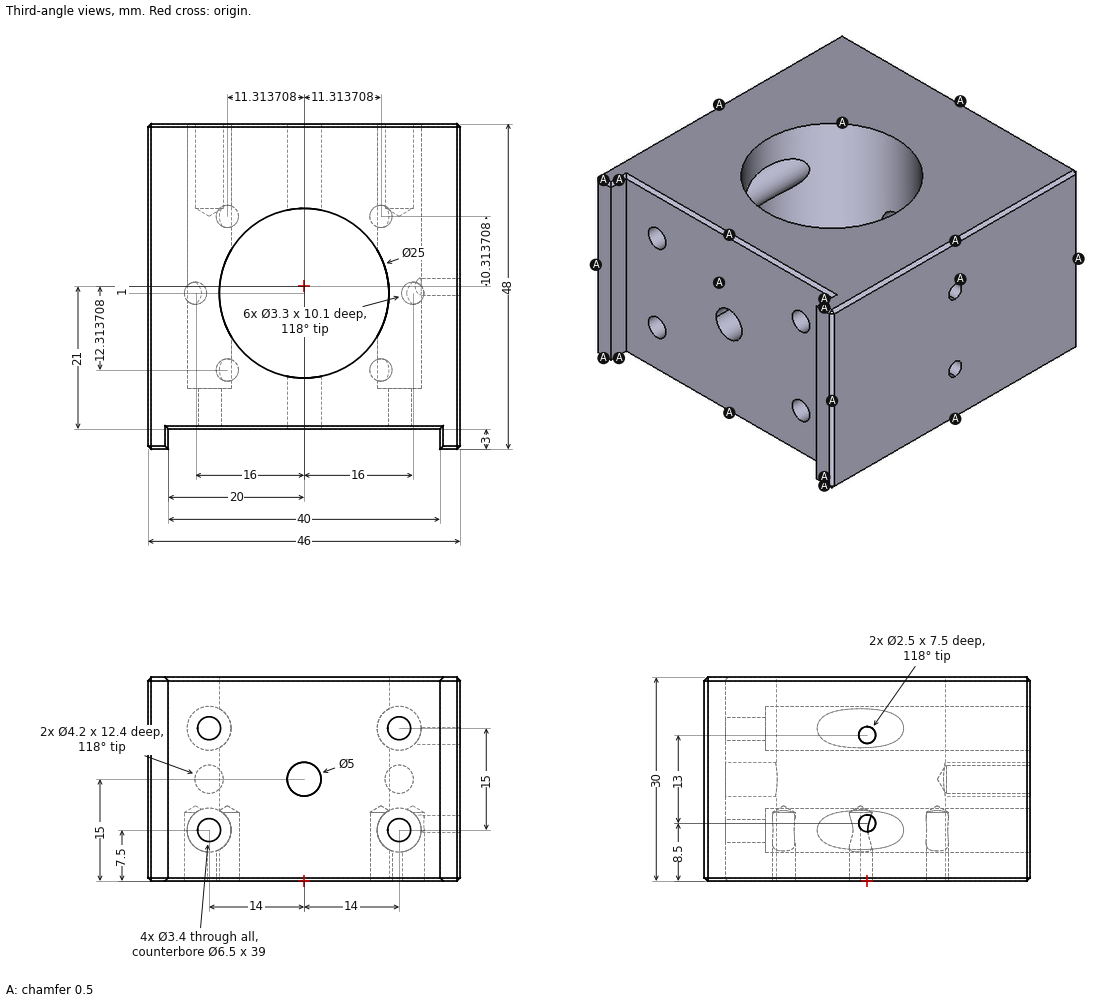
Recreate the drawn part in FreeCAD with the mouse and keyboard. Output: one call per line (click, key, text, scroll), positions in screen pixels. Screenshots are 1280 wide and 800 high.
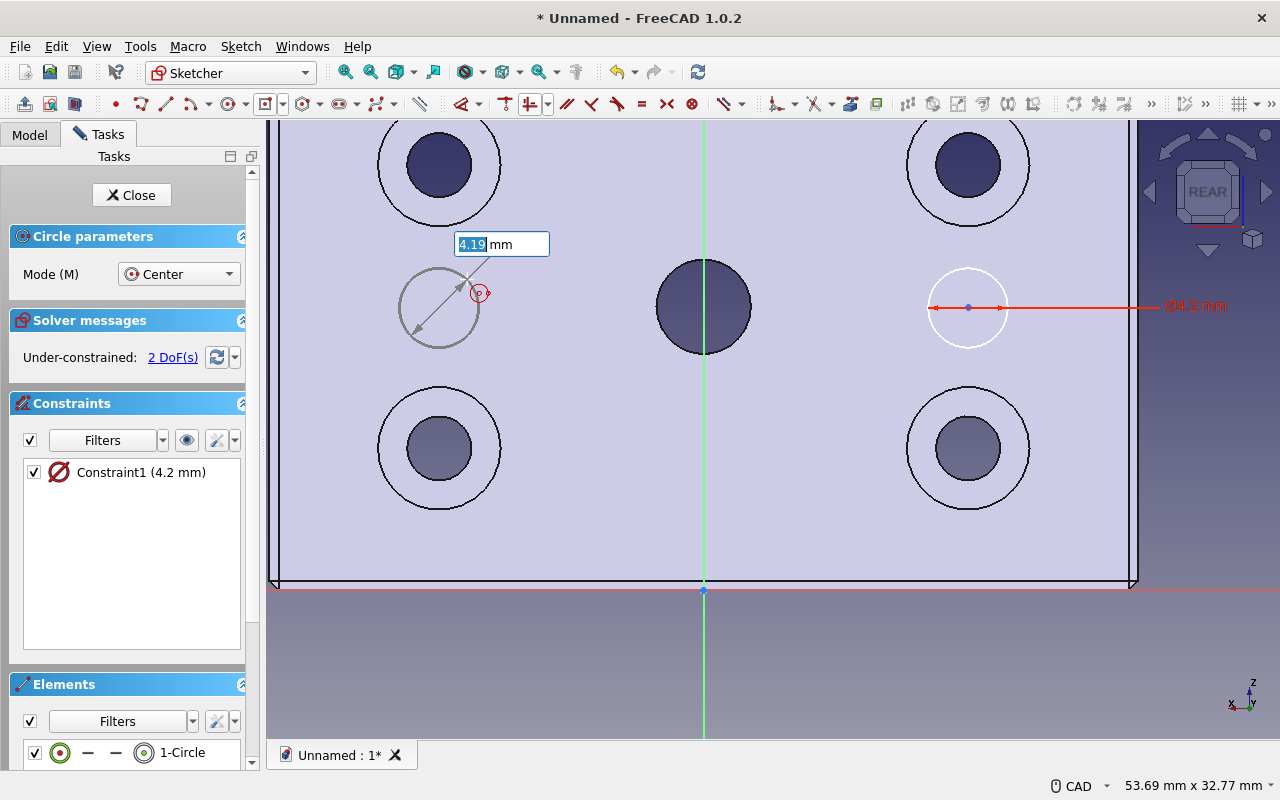
text(4.2)
key(Return)
key(Escape)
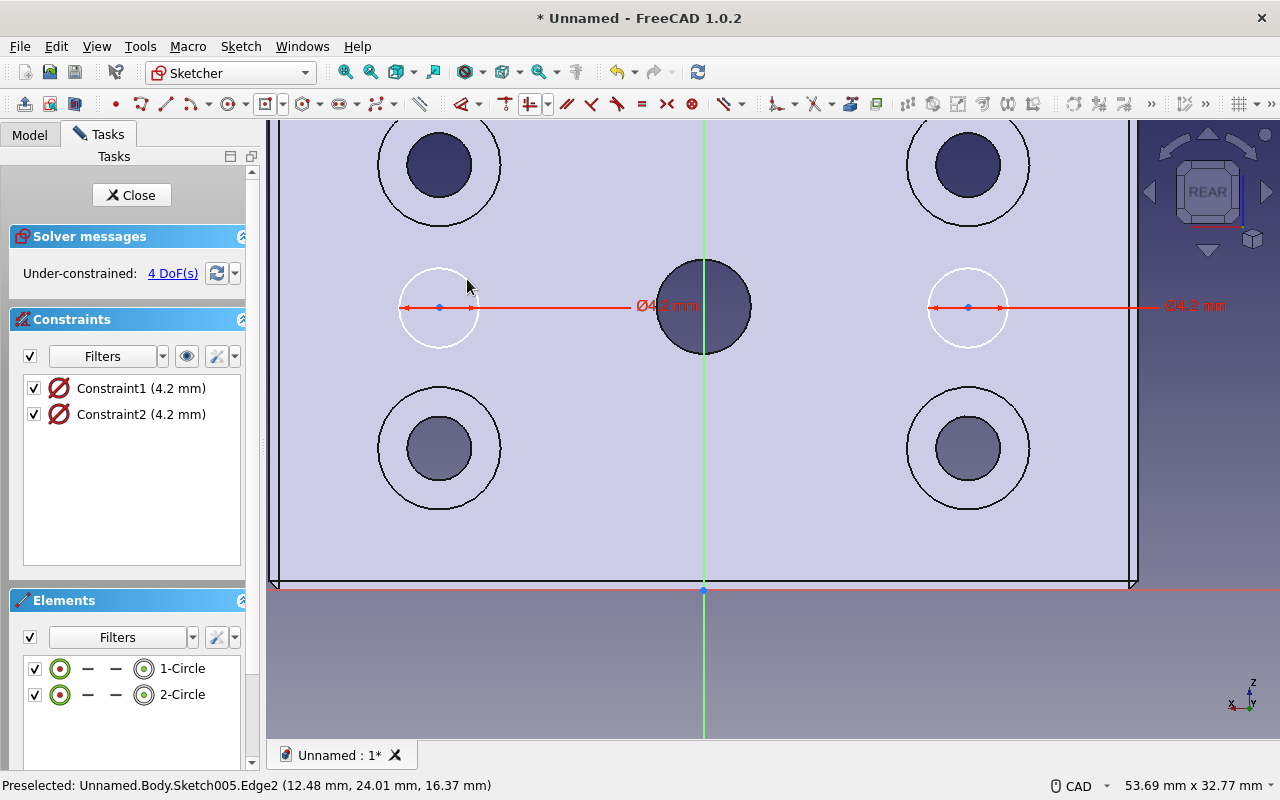
click(968, 308)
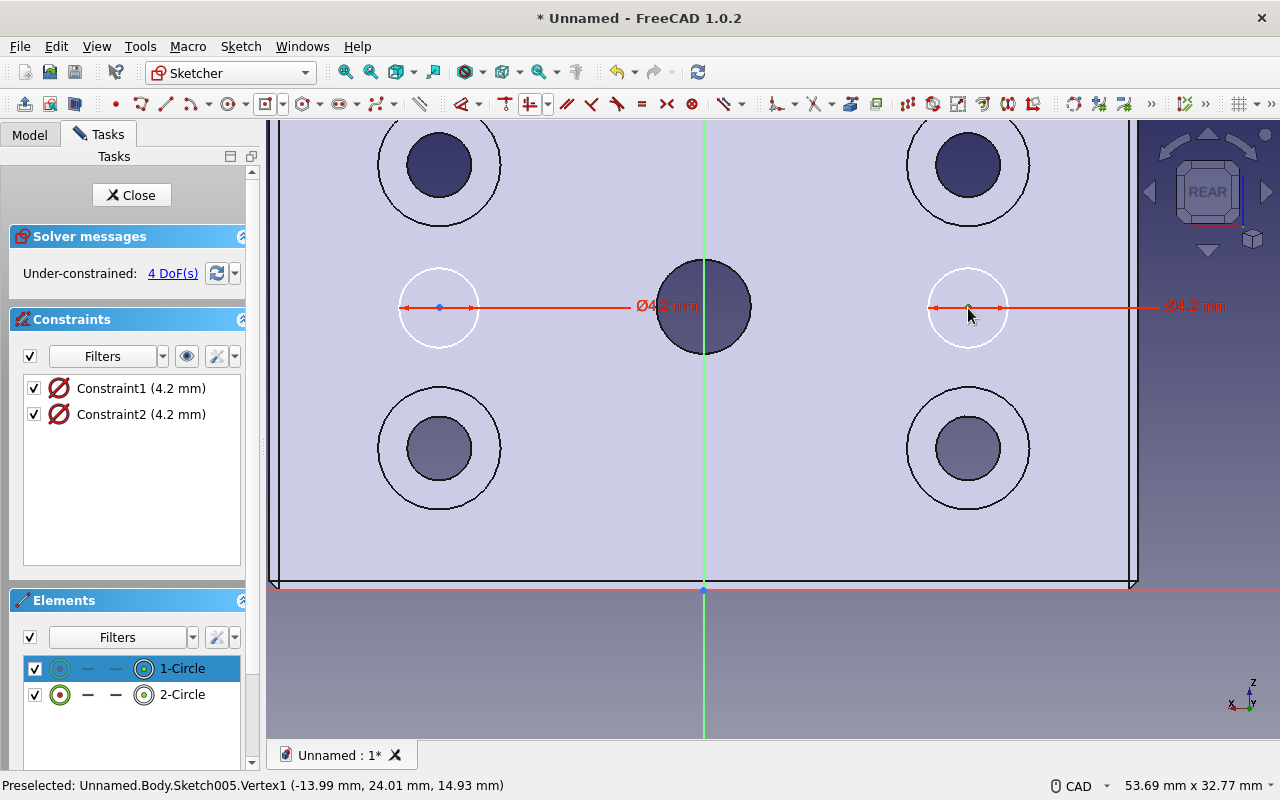
click(439, 308)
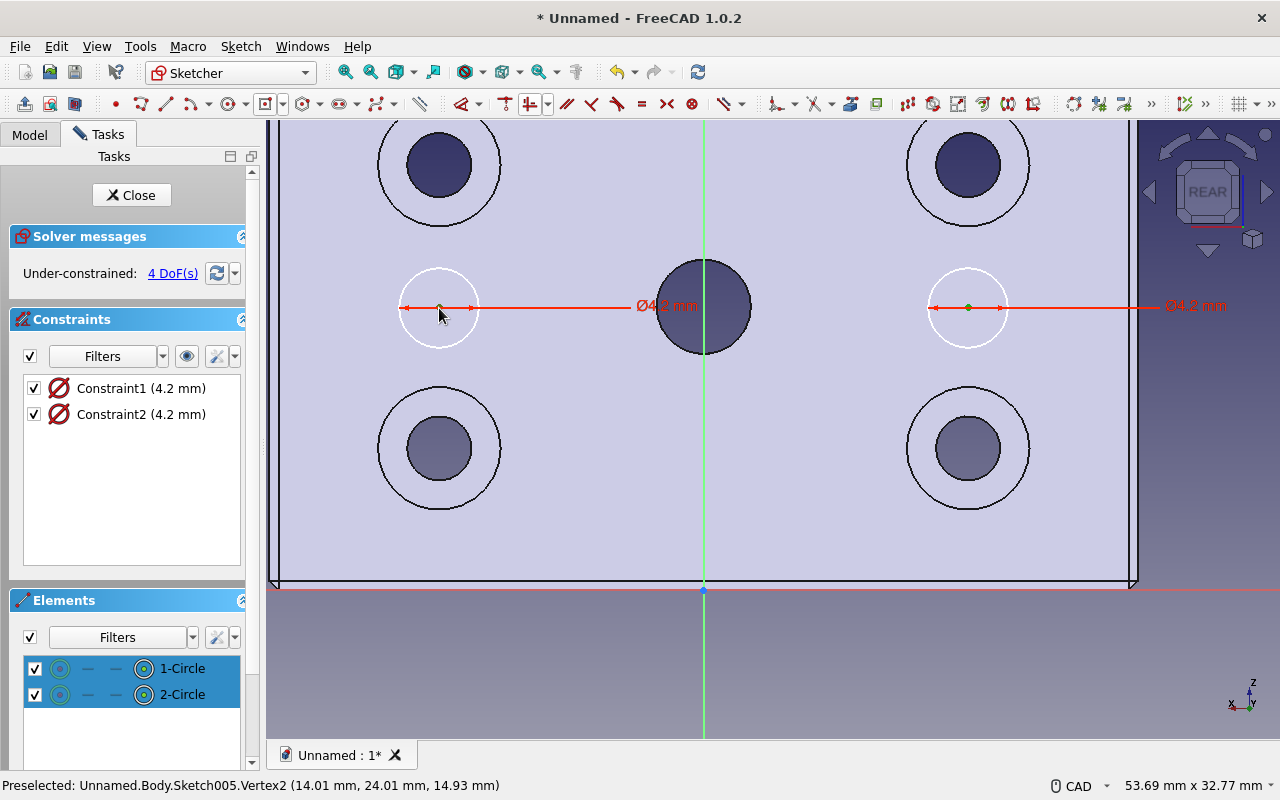
click(548, 104)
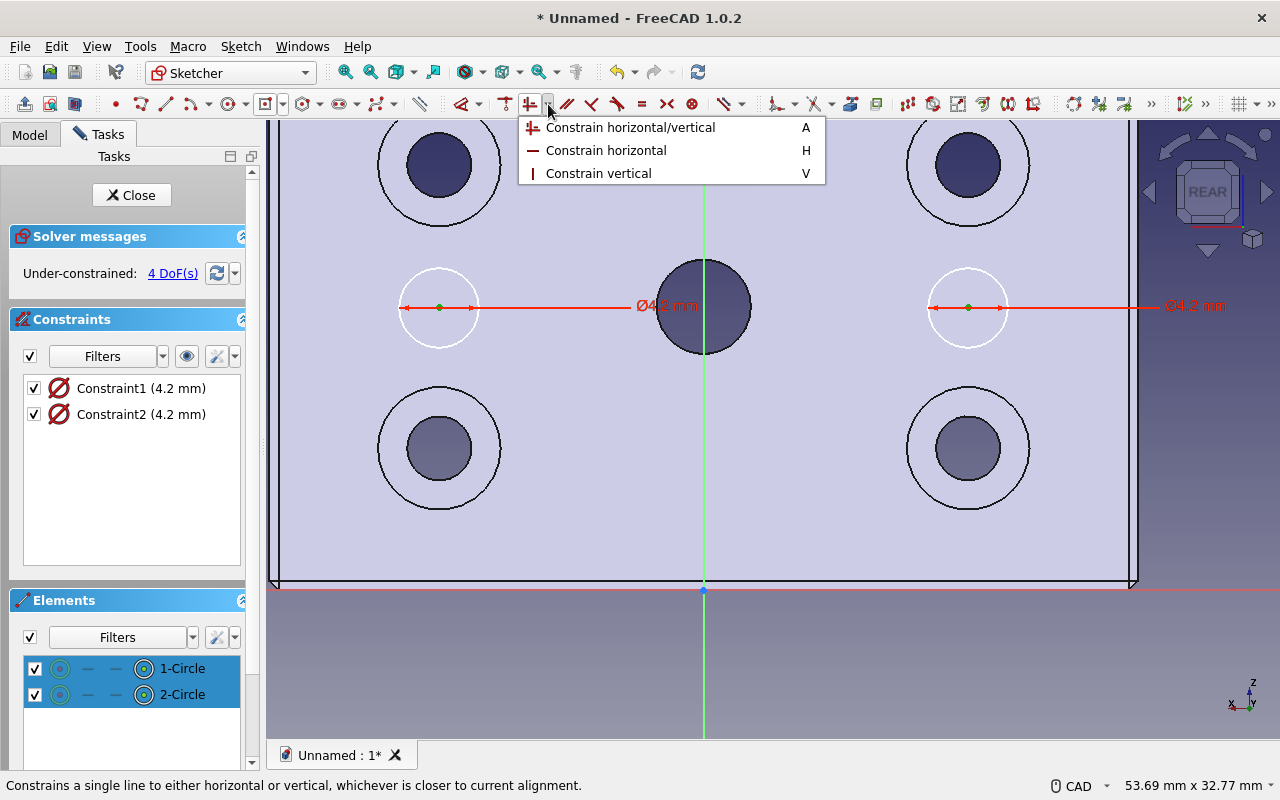
click(672, 150)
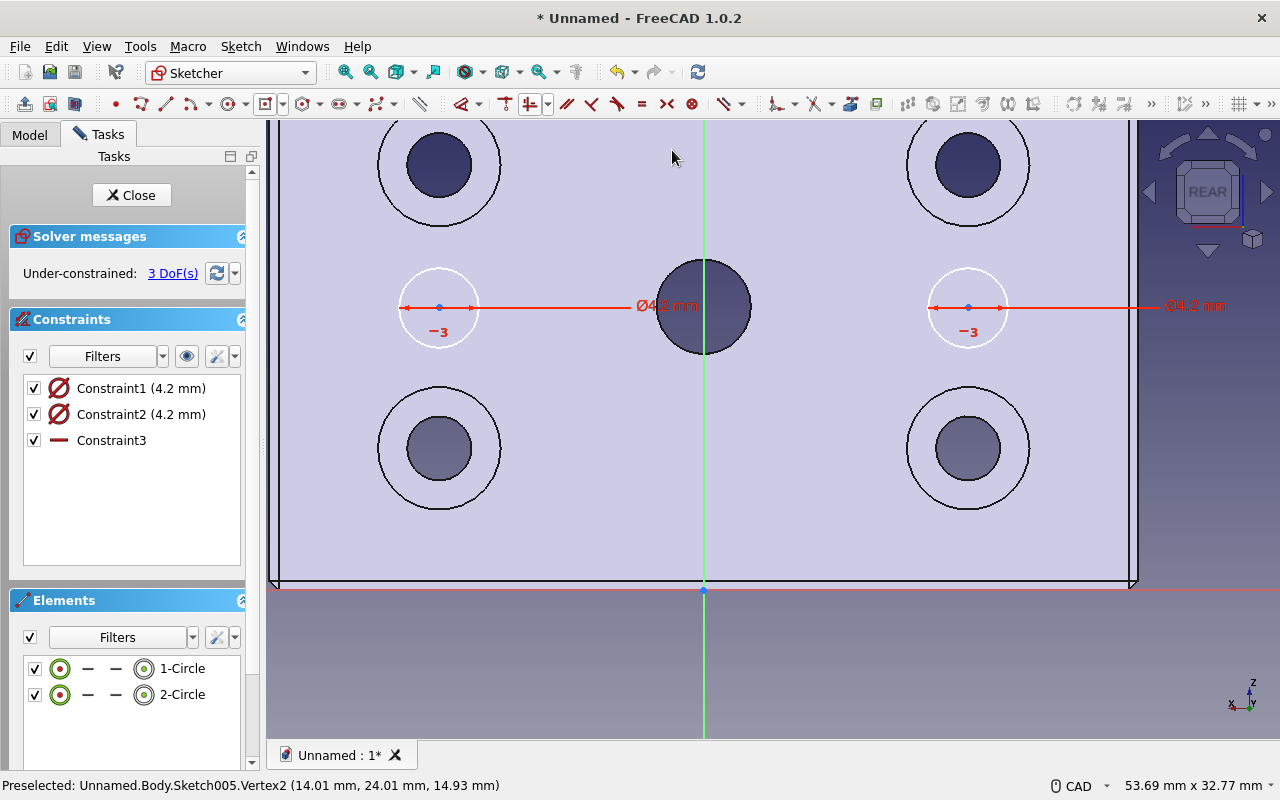
click(460, 104)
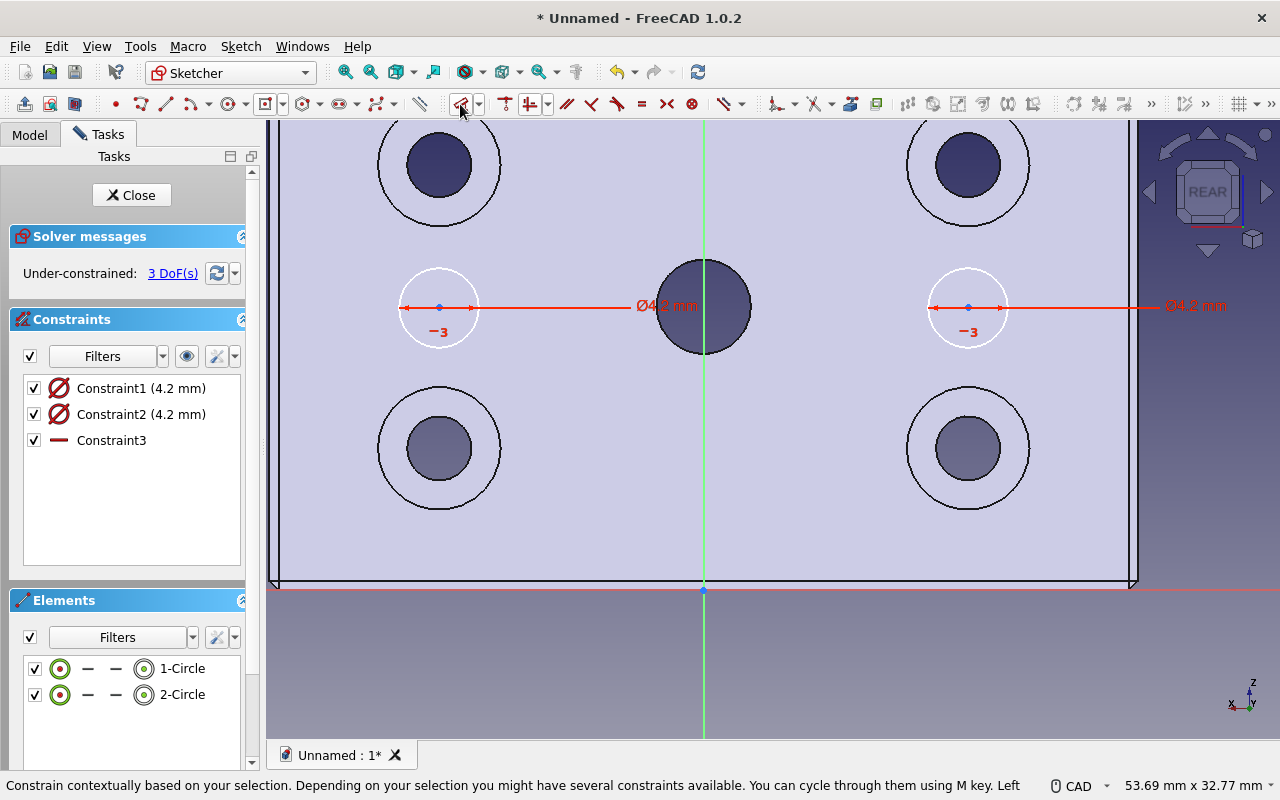
click(968, 308)
click(836, 624)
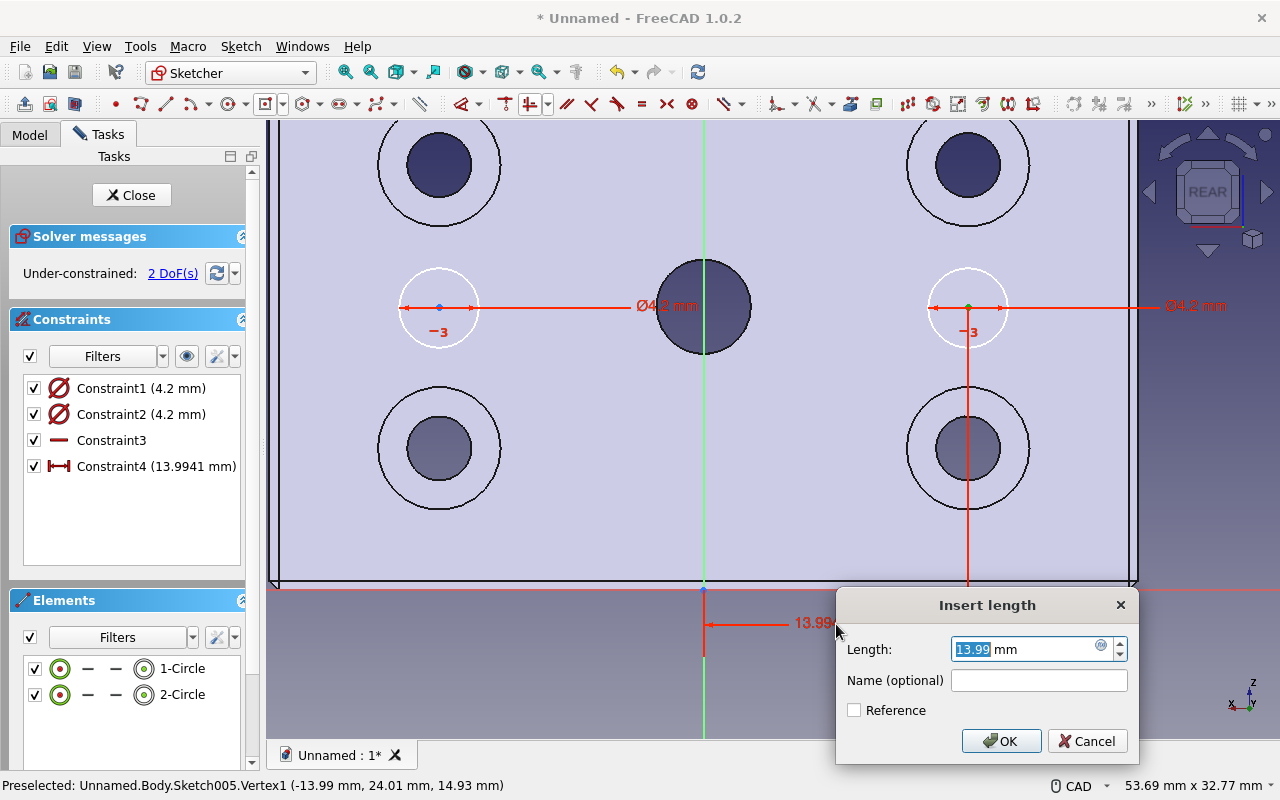
text(14)
key(Return)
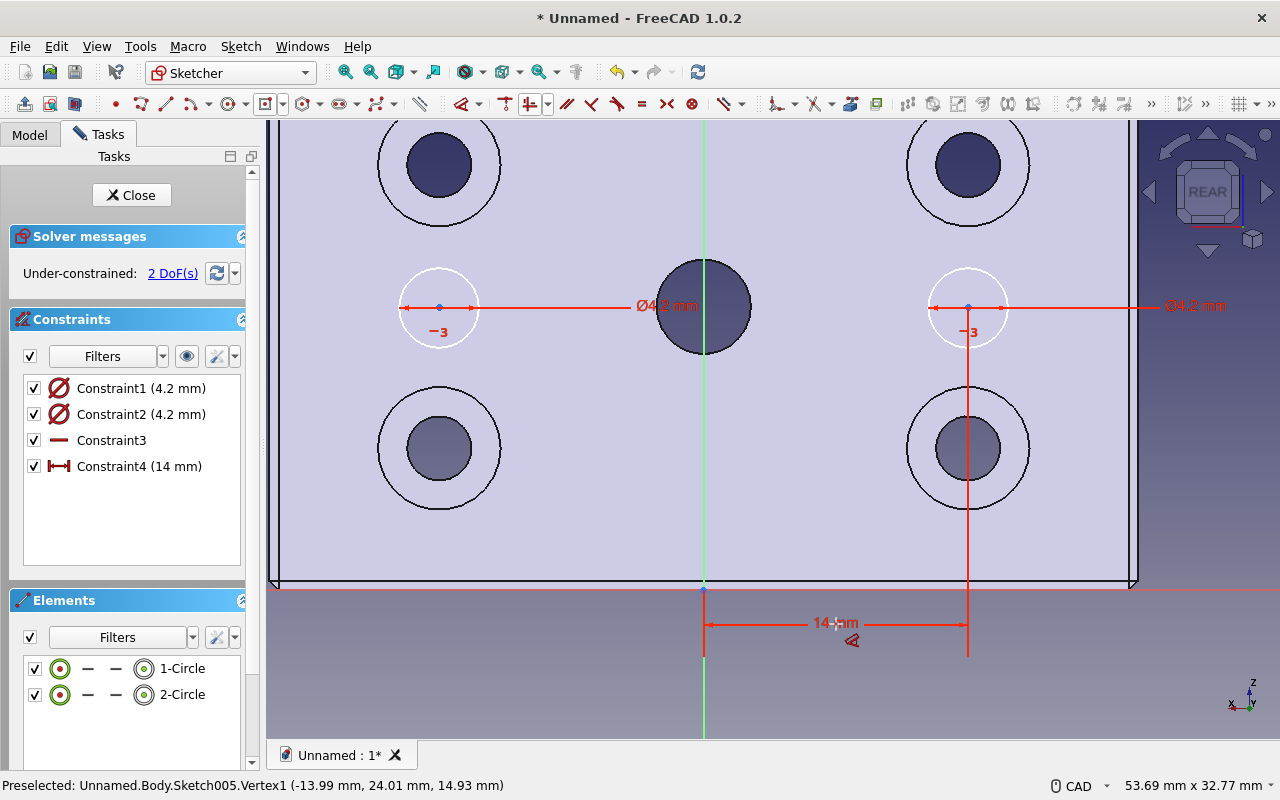
click(968, 308)
click(1002, 449)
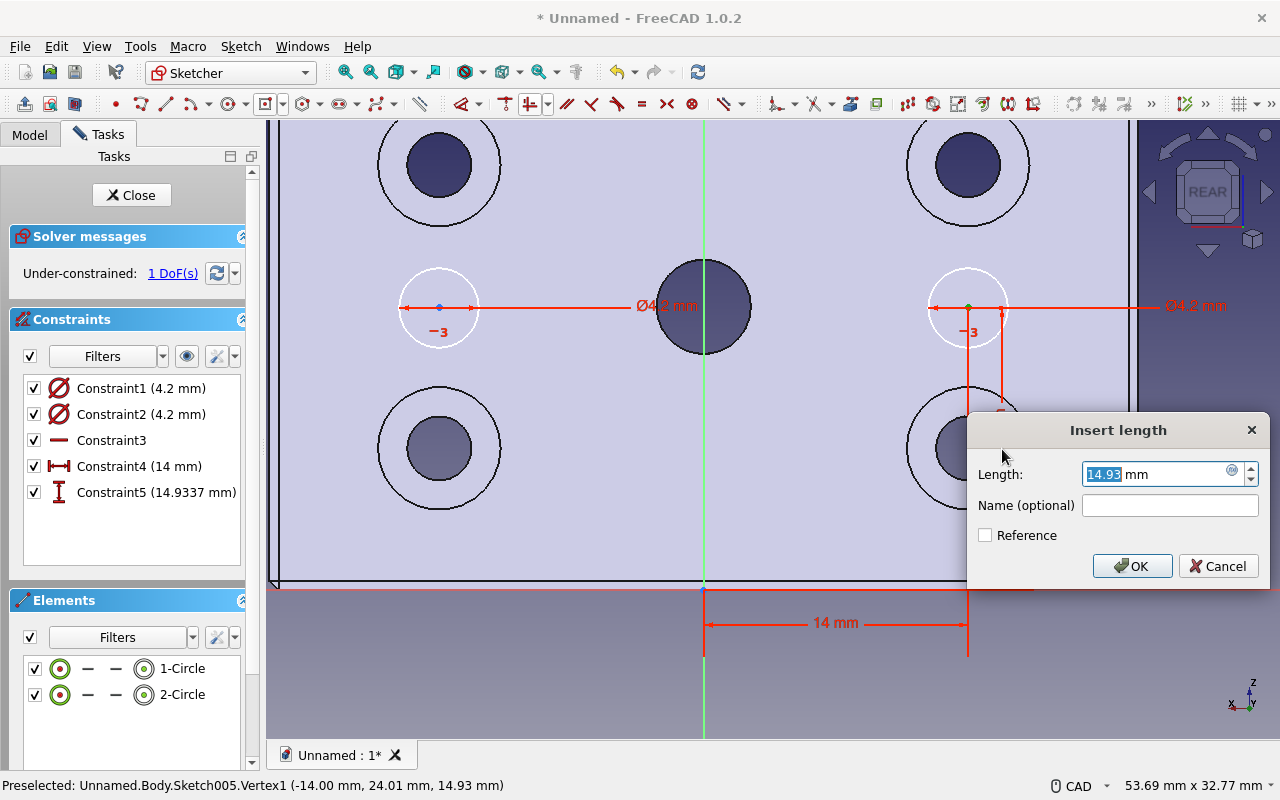
text(15)
key(Return)